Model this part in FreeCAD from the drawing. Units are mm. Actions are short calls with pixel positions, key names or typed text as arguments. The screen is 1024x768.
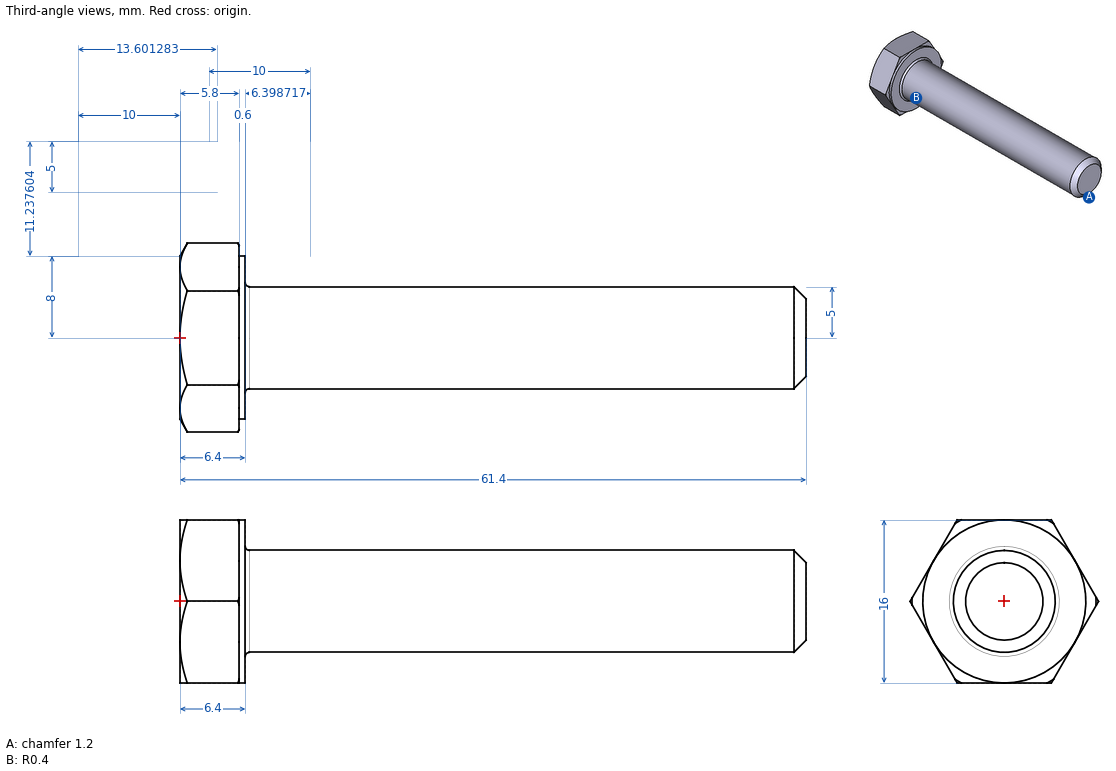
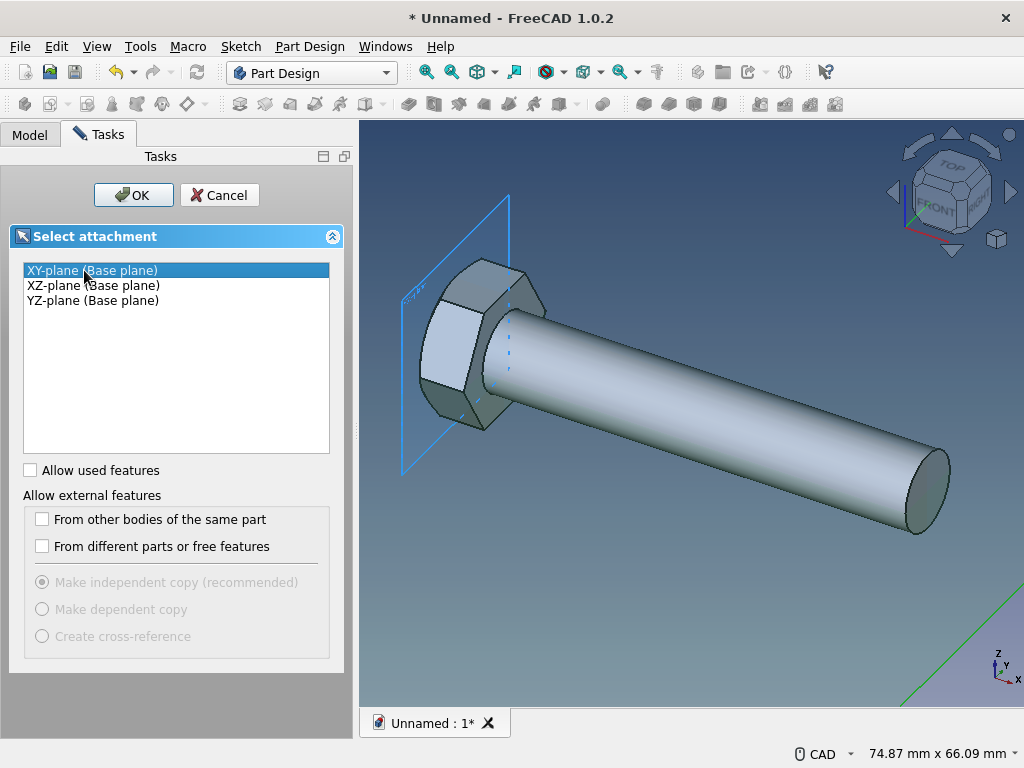
click(134, 195)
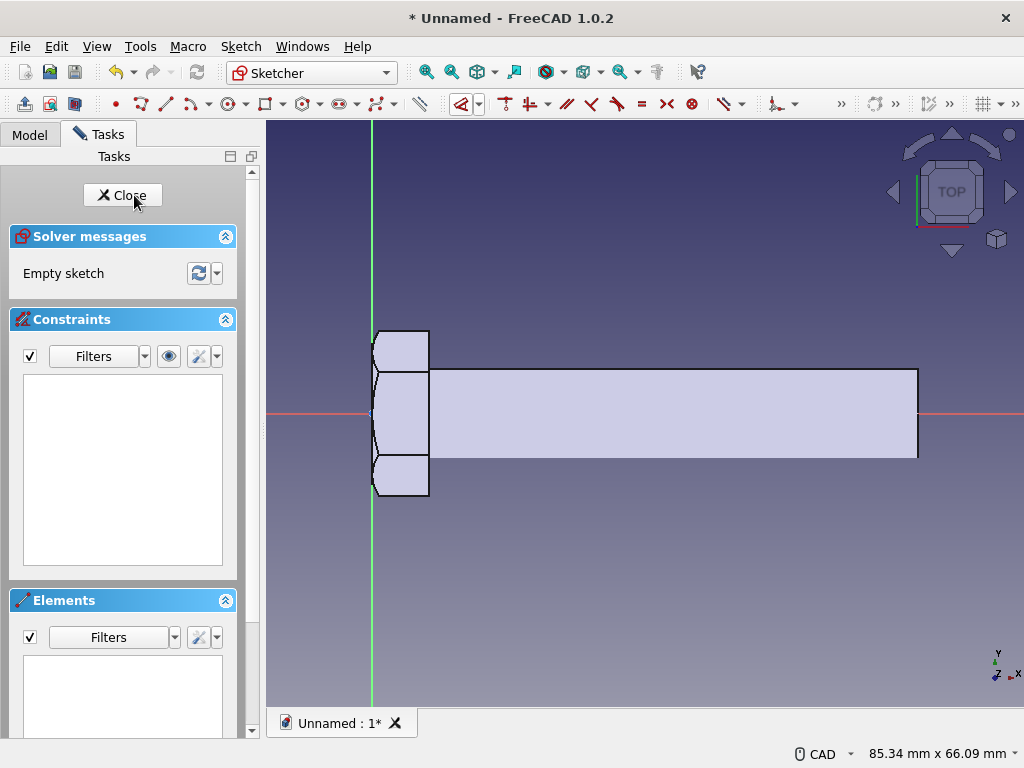
click(75, 104)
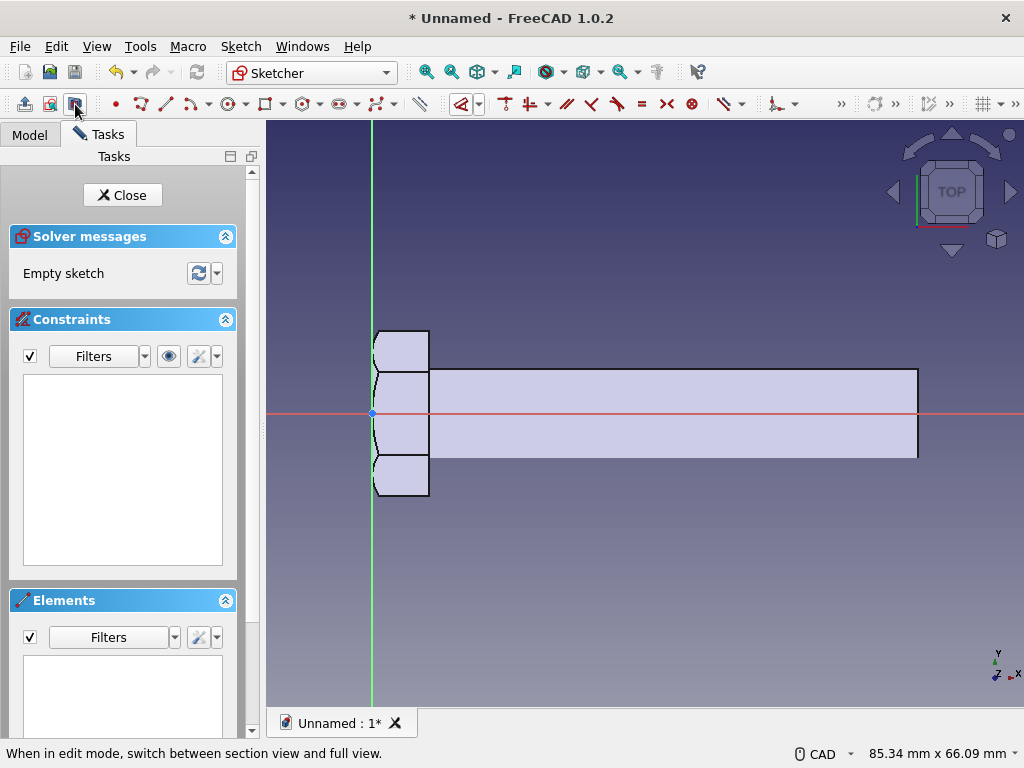
scroll(309, 258, up, 4)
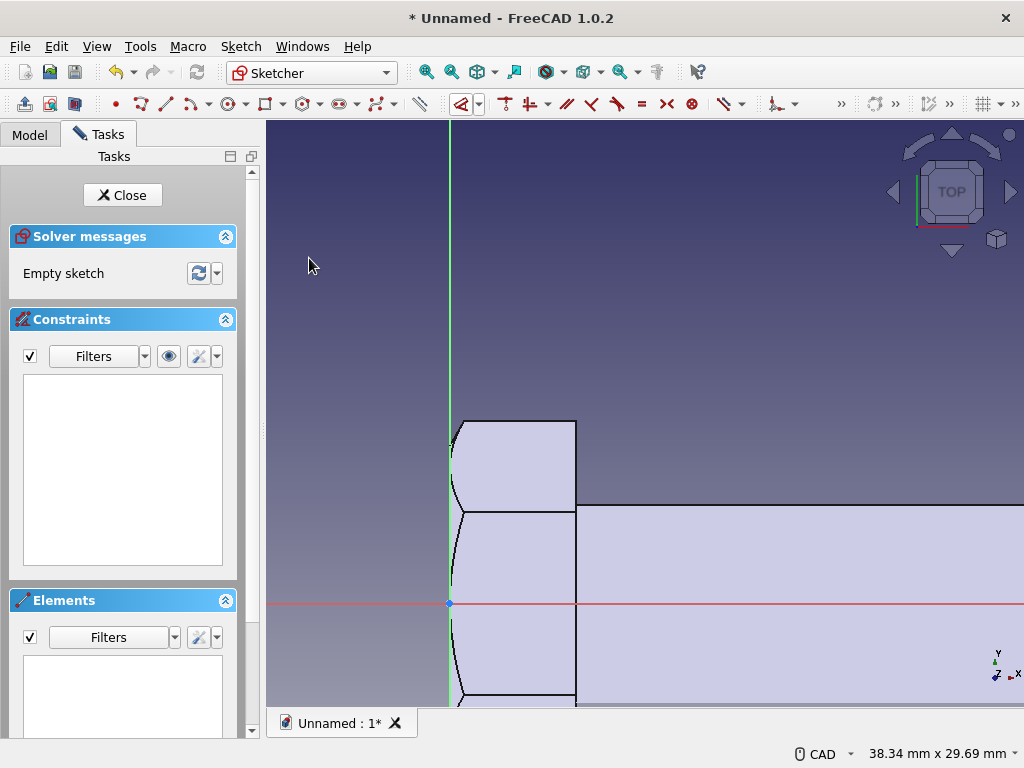
click(141, 104)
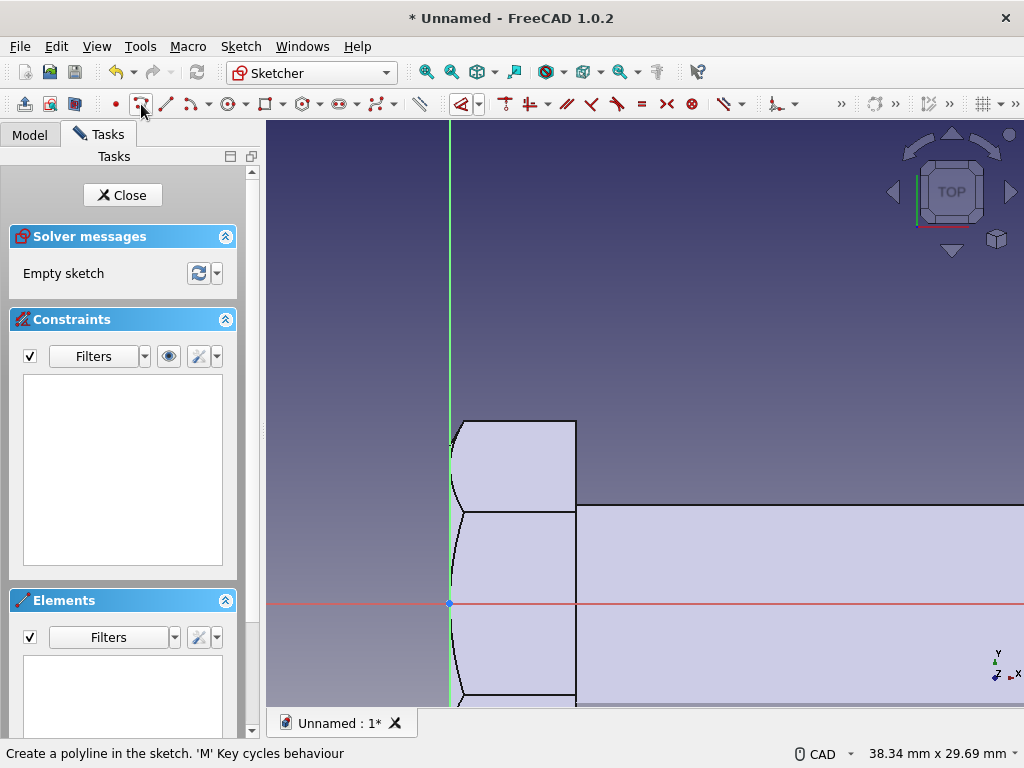
click(576, 446)
click(703, 446)
click(703, 223)
click(505, 223)
click(505, 322)
click(576, 447)
key(Escape)
key(Escape)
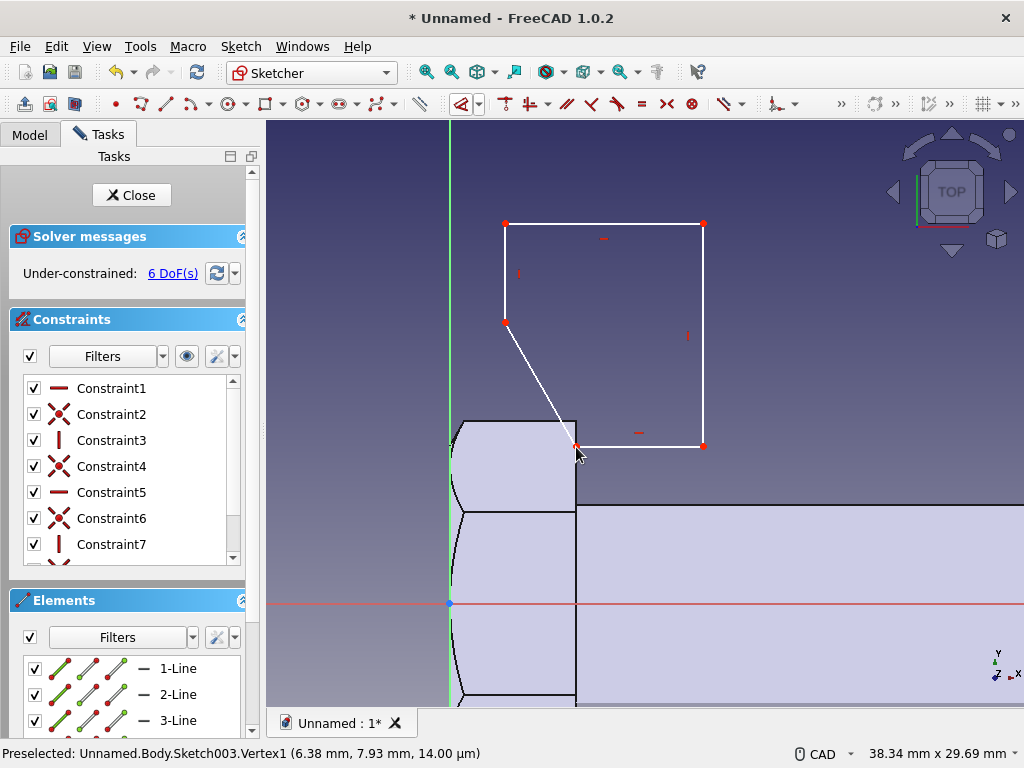
click(505, 254)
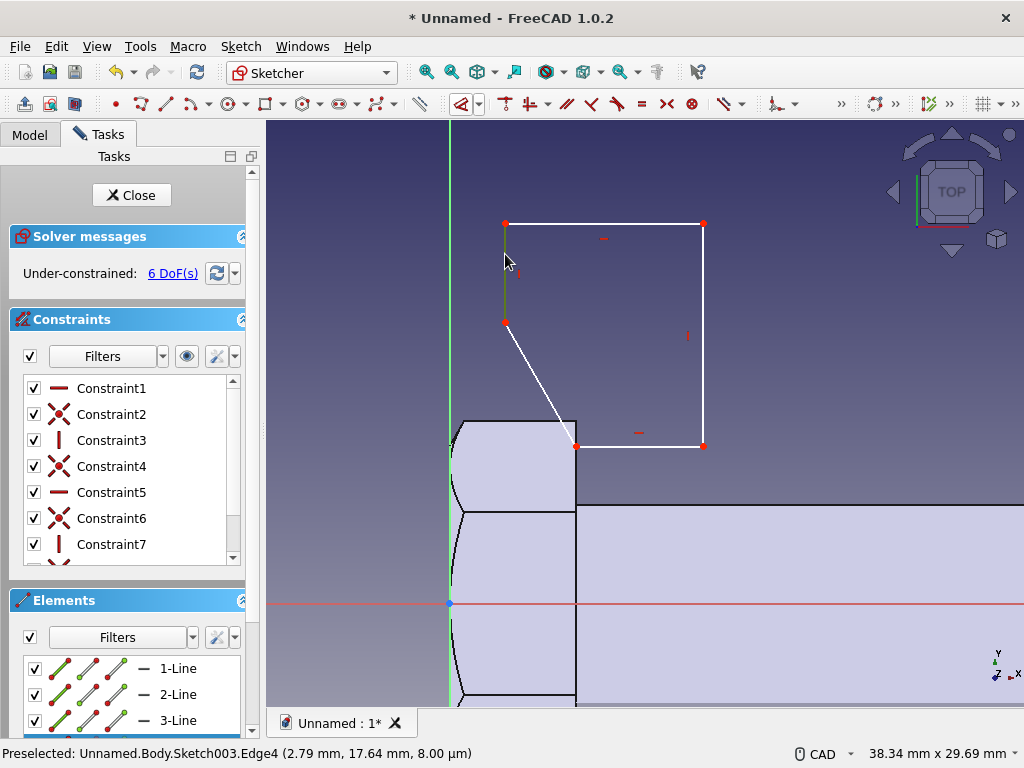
key(i)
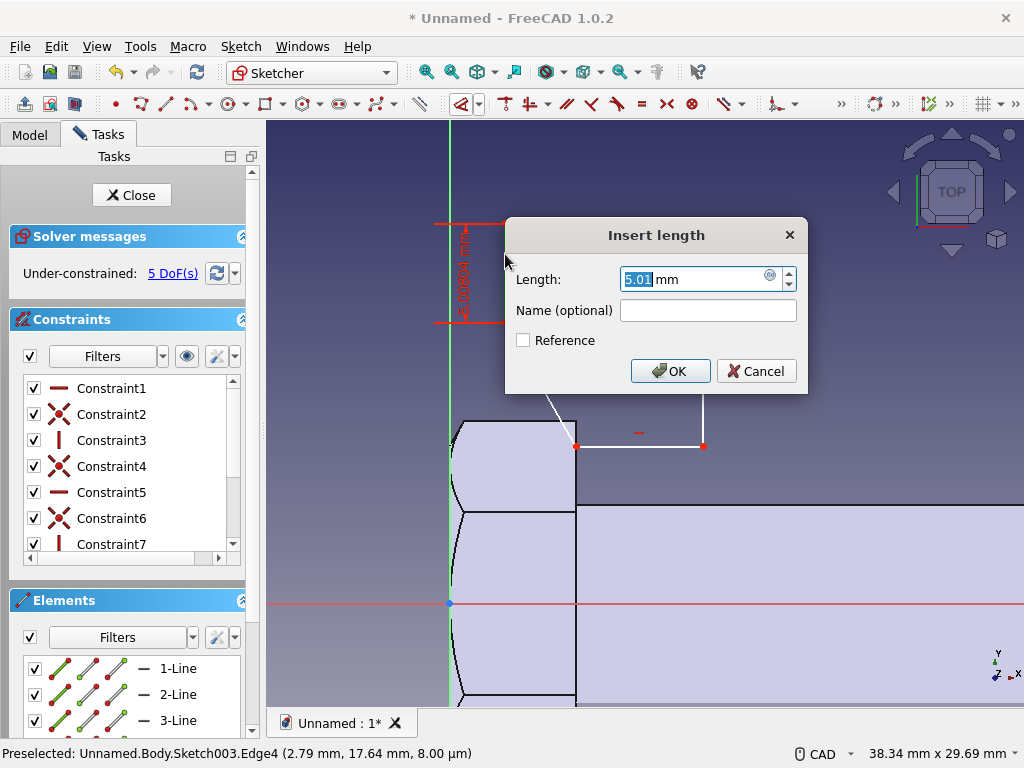
text(5)
key(Return)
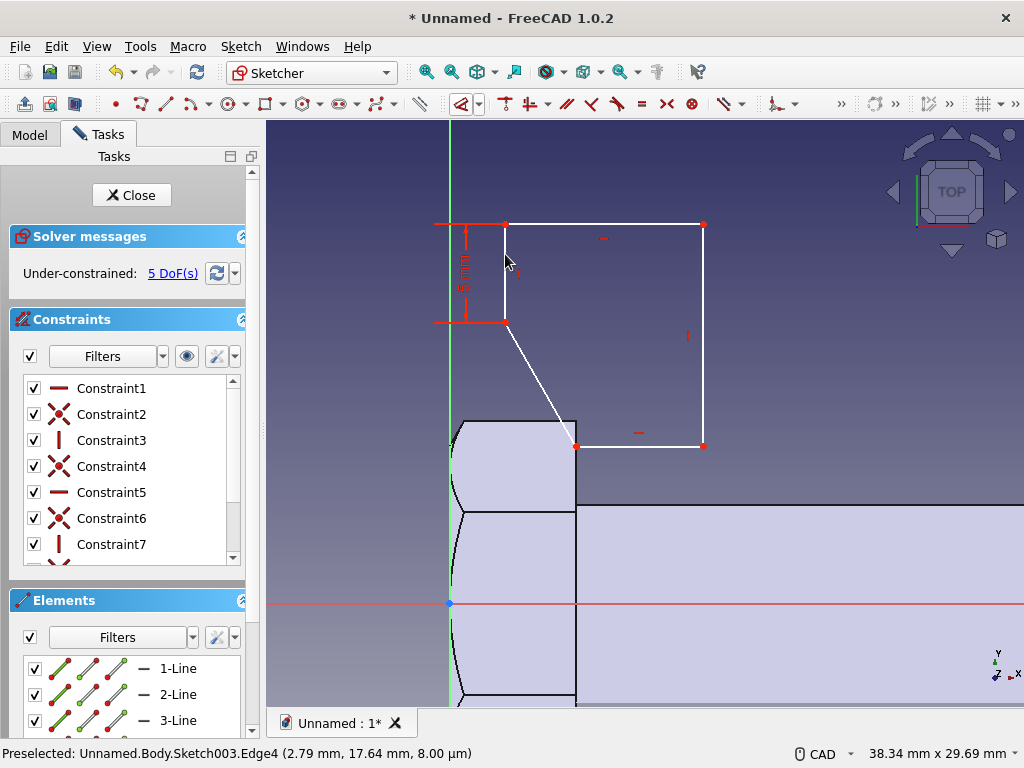
click(644, 224)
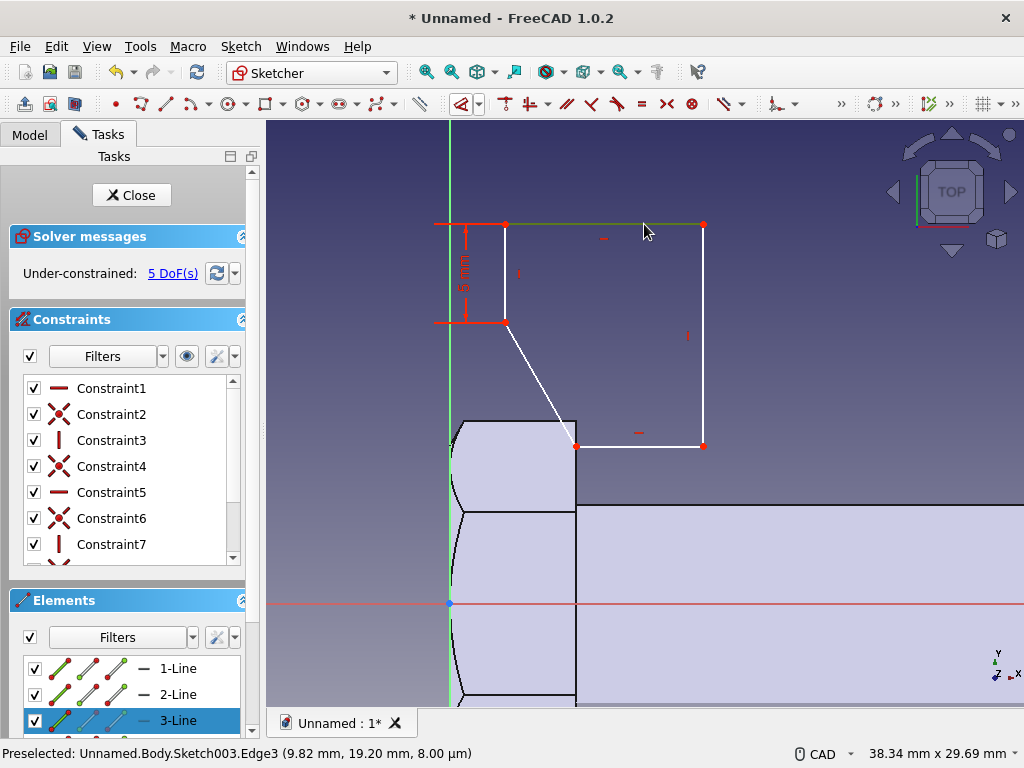
click(478, 104)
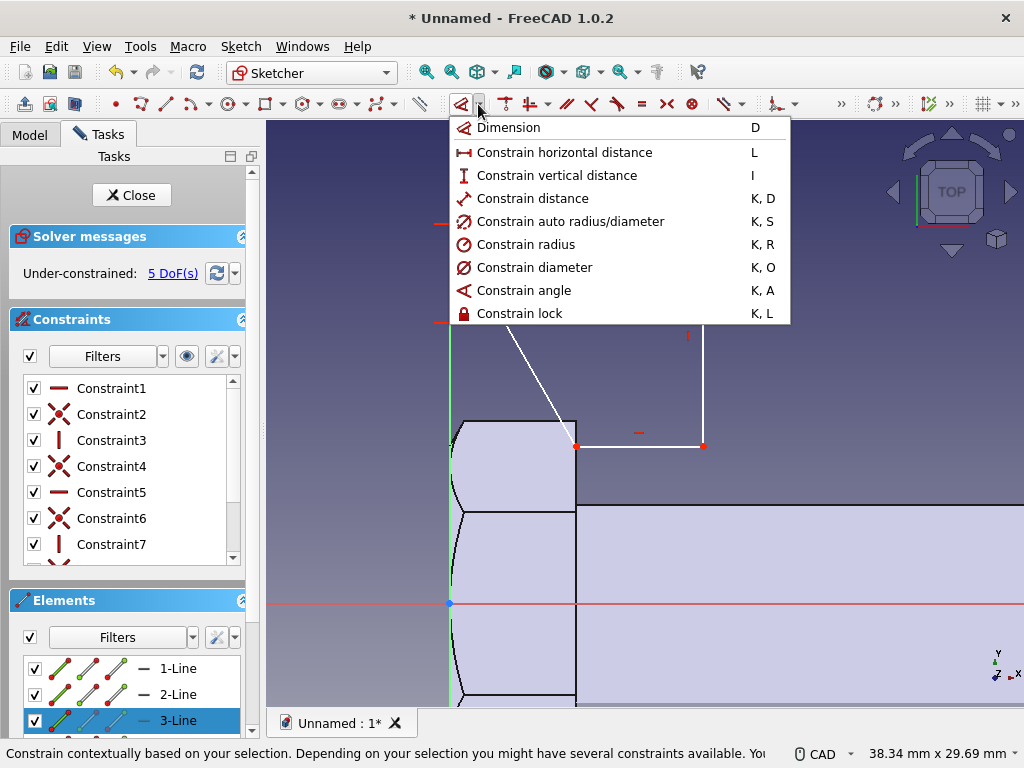
click(620, 152)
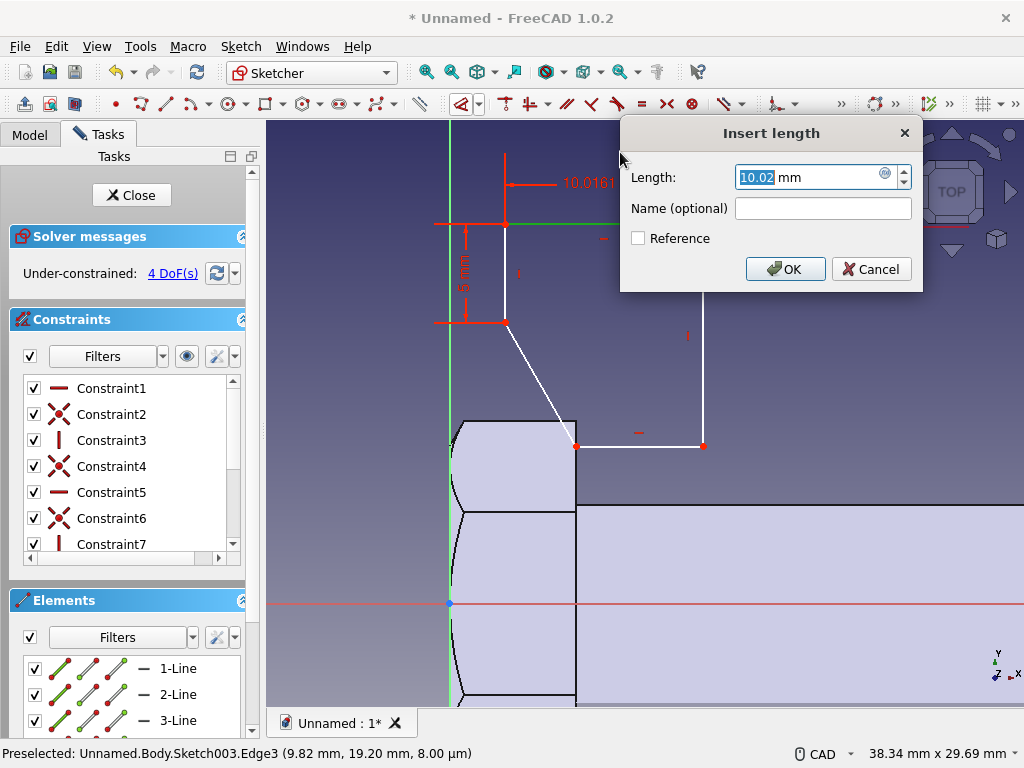
text(10)
key(Return)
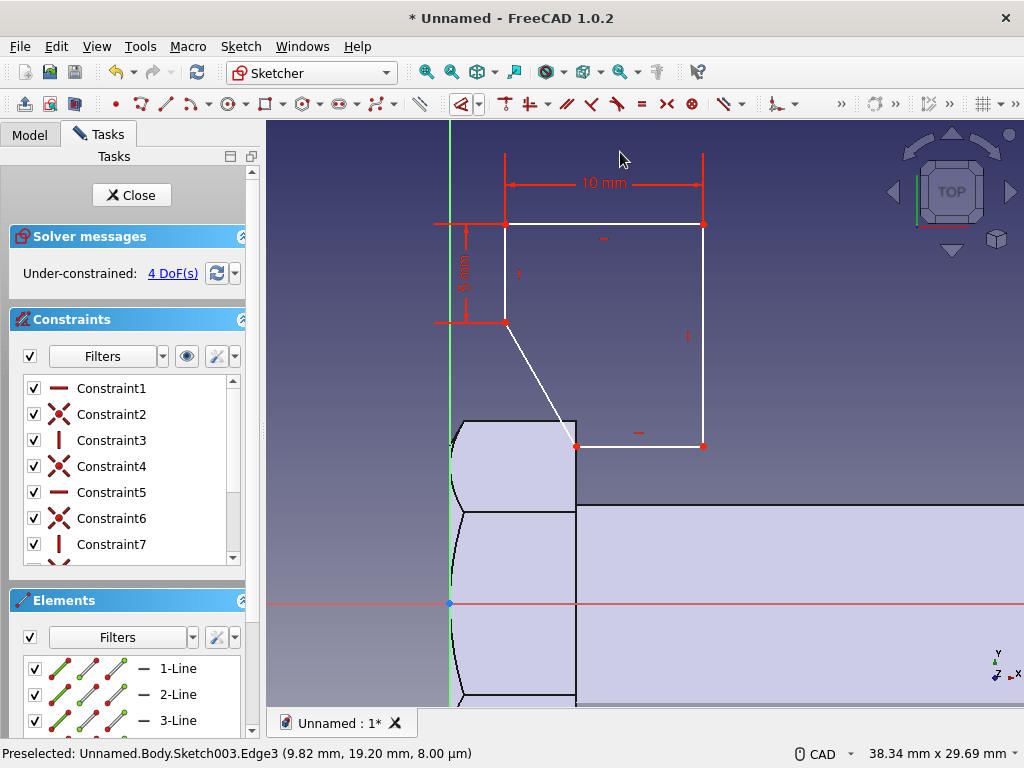
click(576, 447)